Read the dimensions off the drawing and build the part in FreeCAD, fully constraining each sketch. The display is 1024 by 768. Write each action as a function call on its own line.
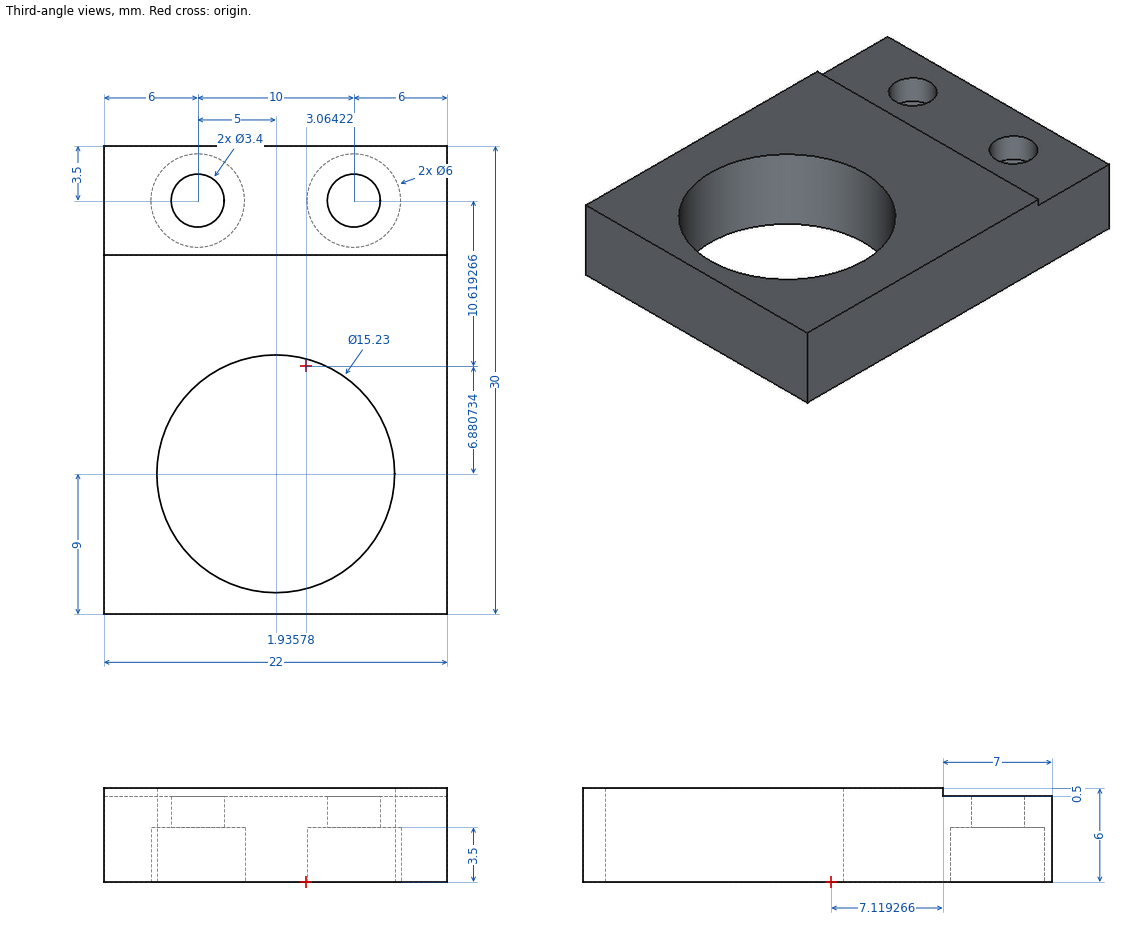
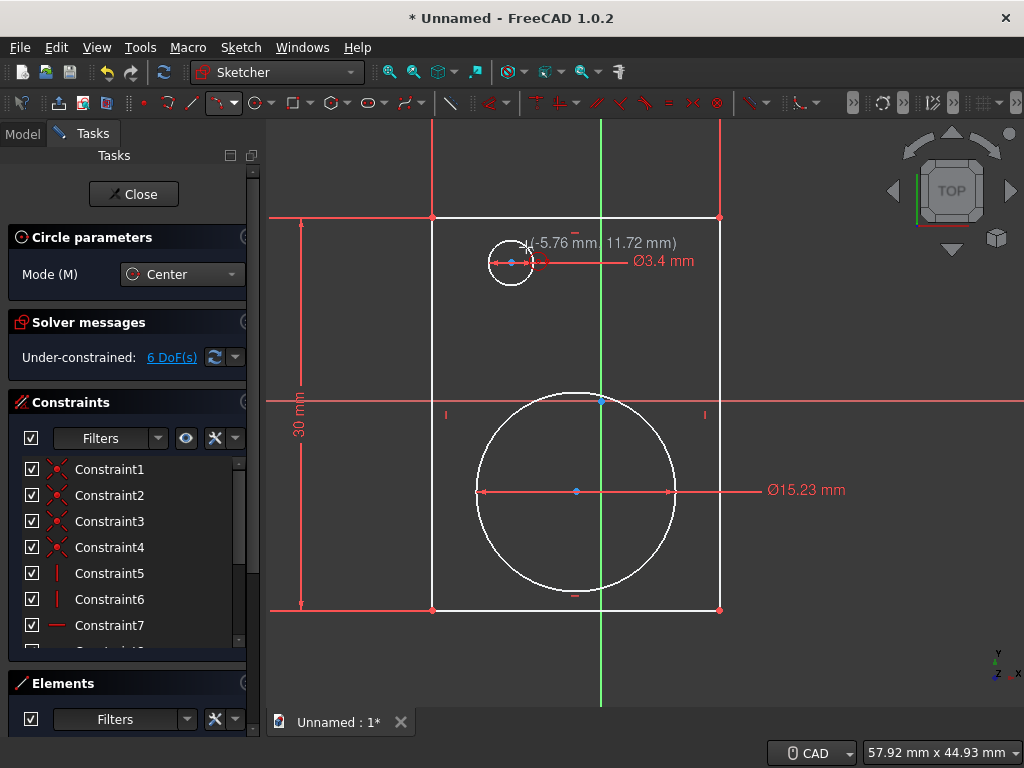
click(642, 262)
move(657, 247)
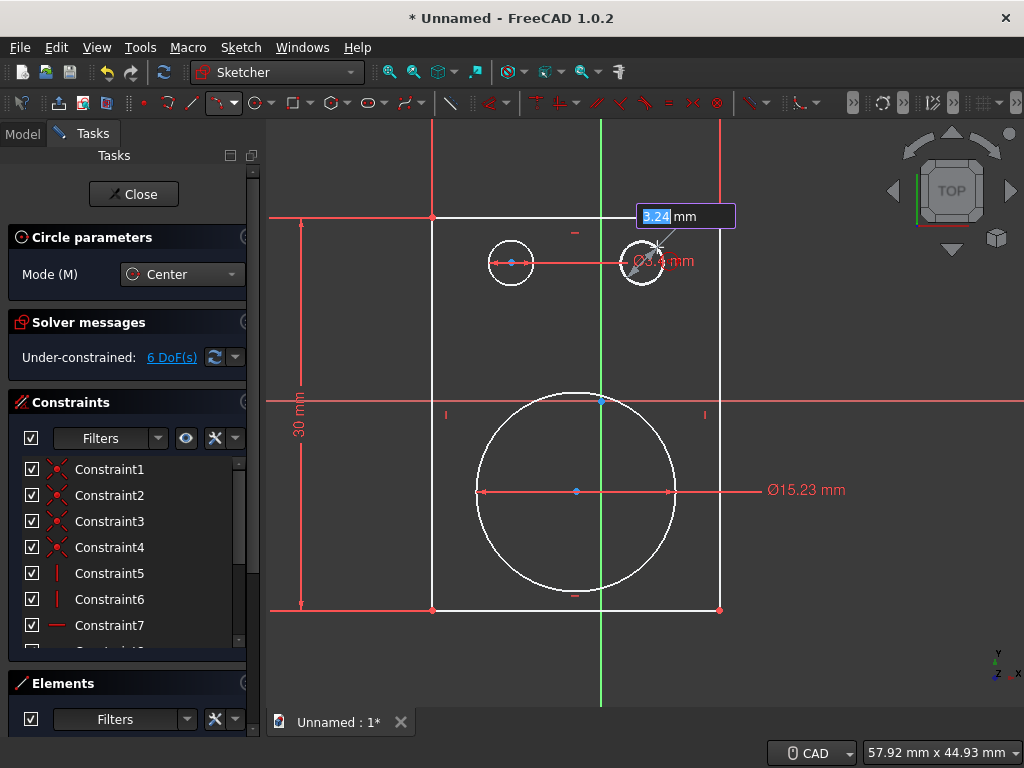
text(3.4)
key(Return)
key(Escape)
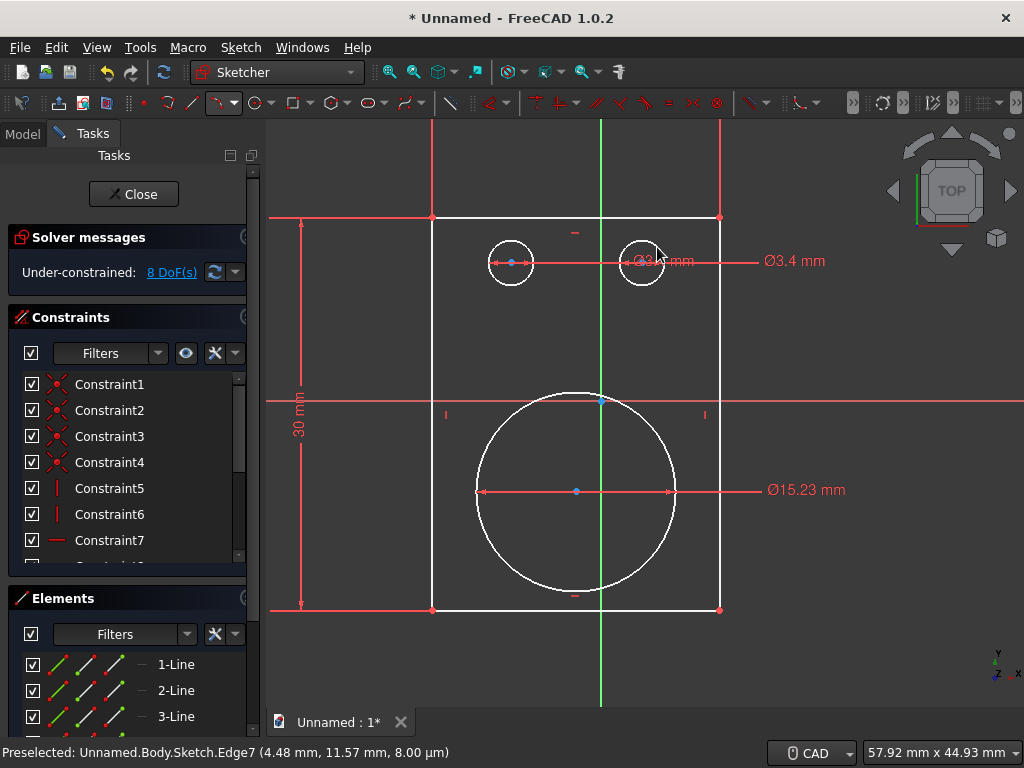
click(511, 263)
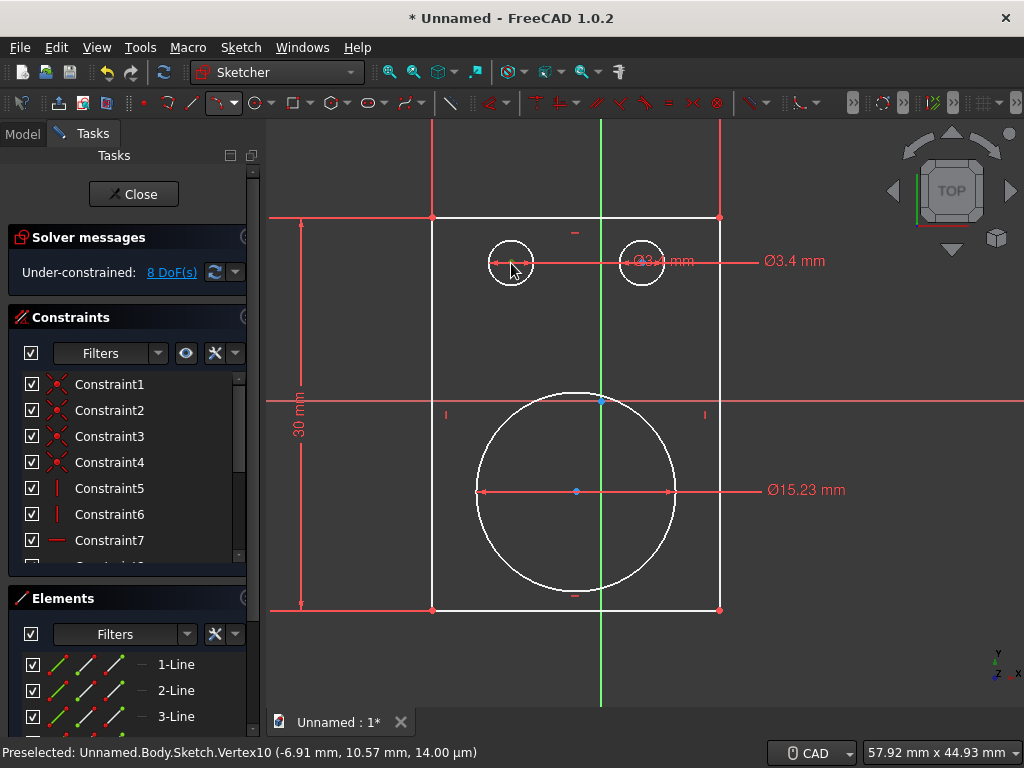
click(642, 263)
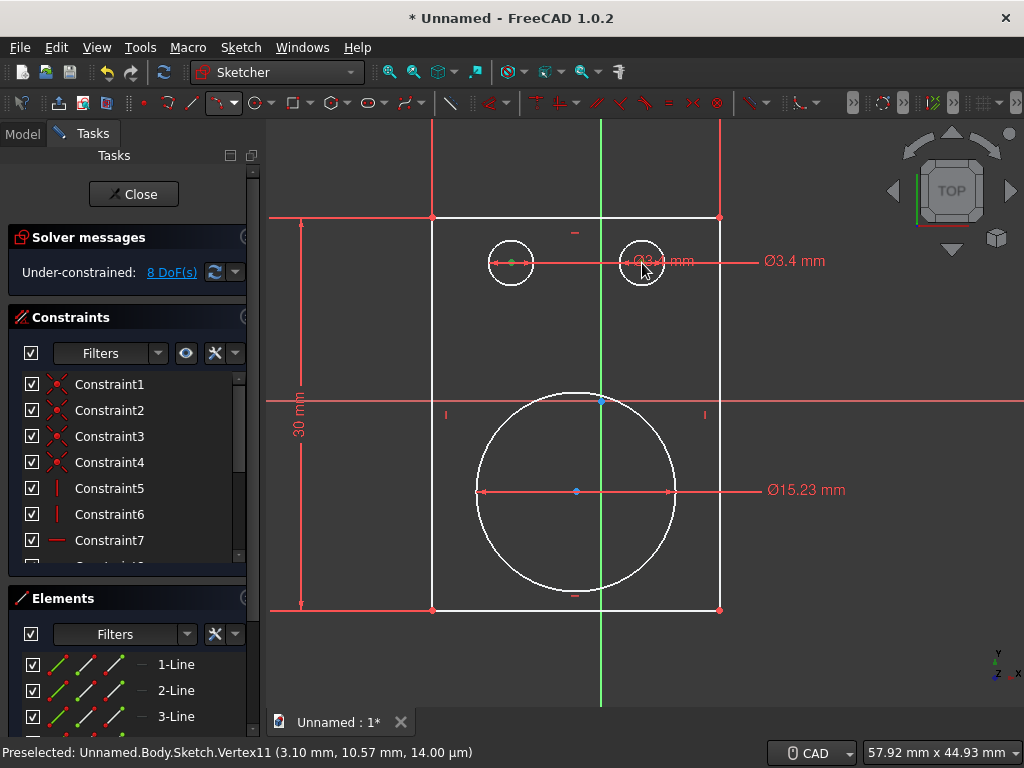
key(h)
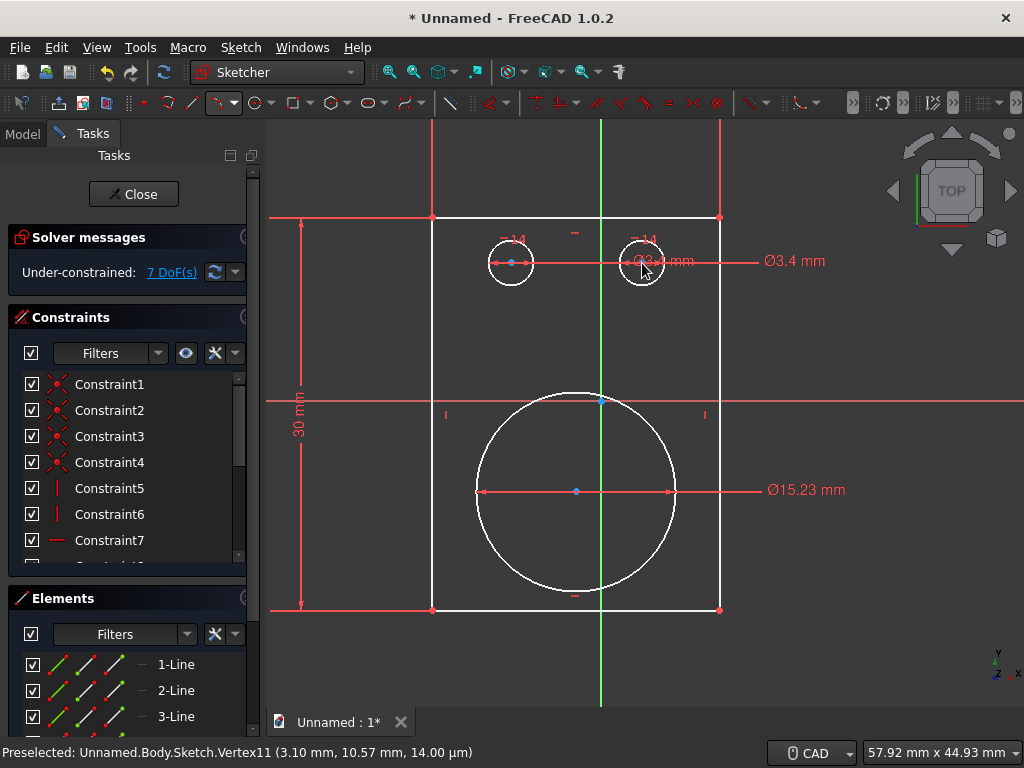
click(432, 611)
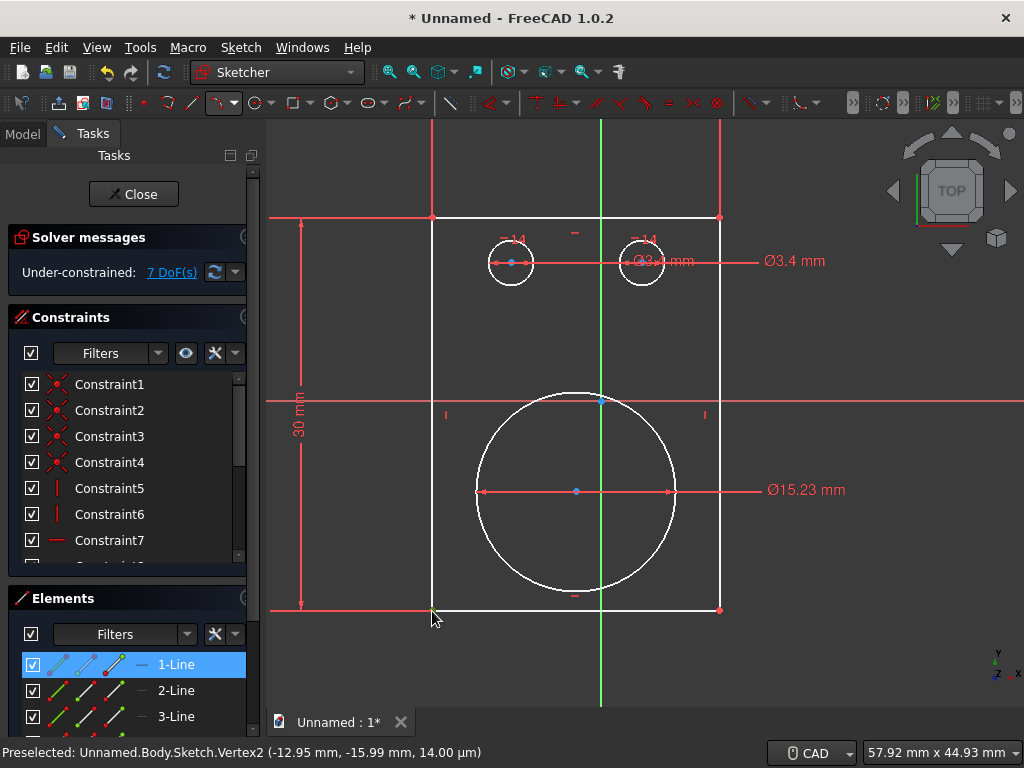
click(576, 492)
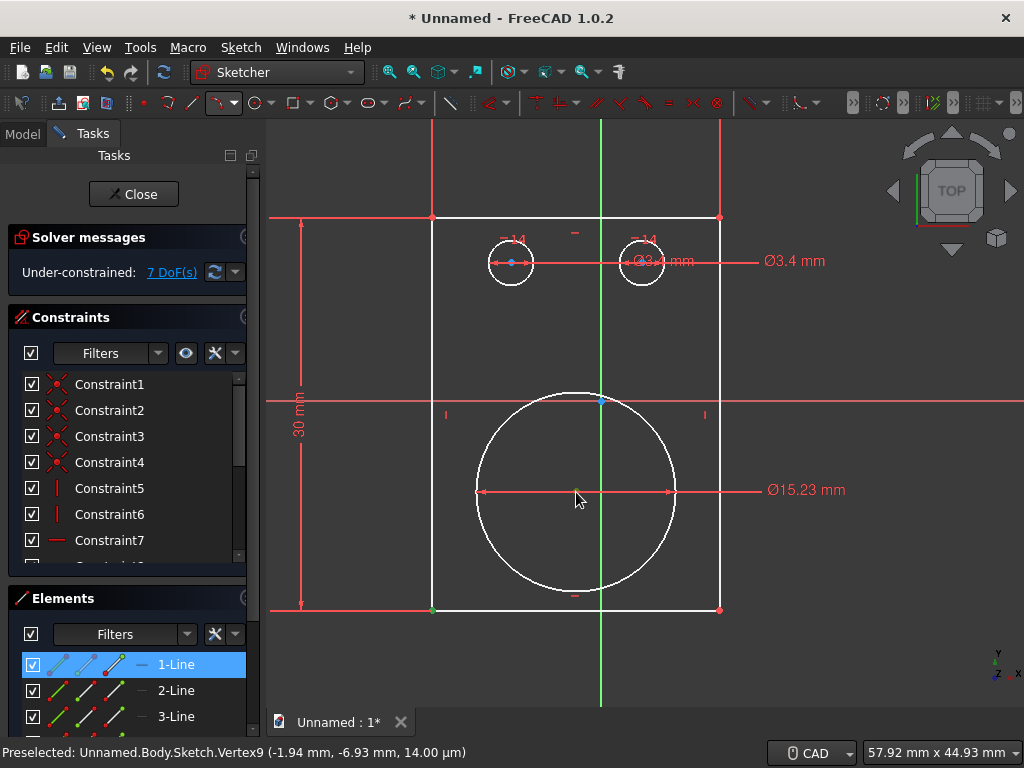
key(i)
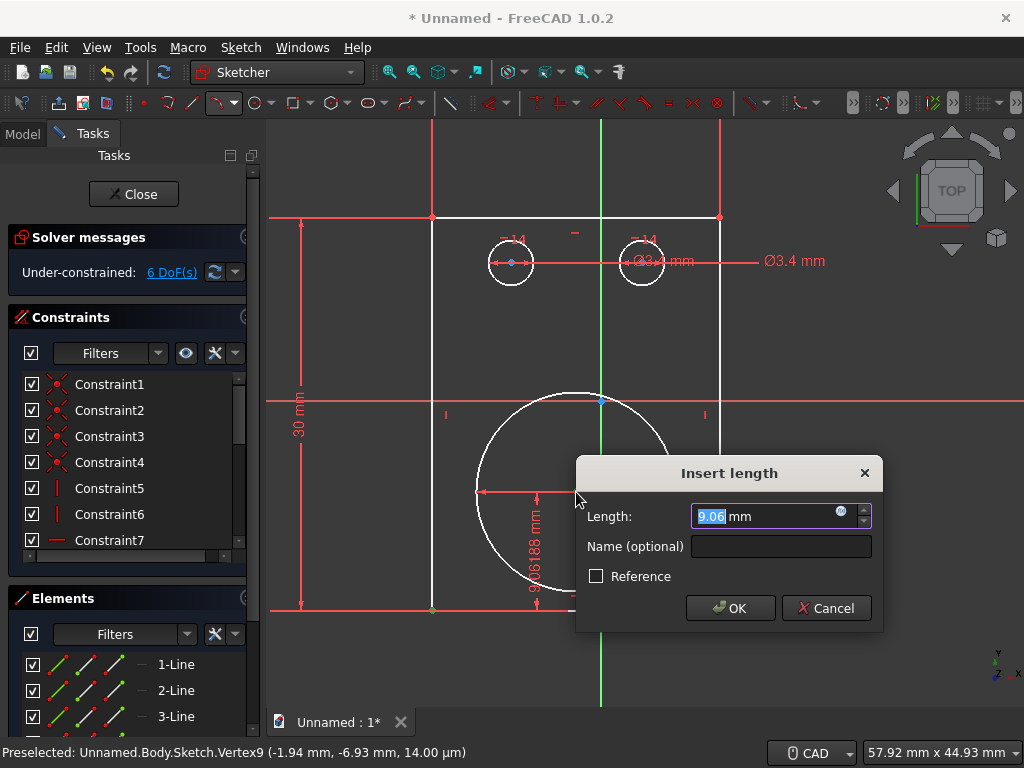
text(9)
key(Return)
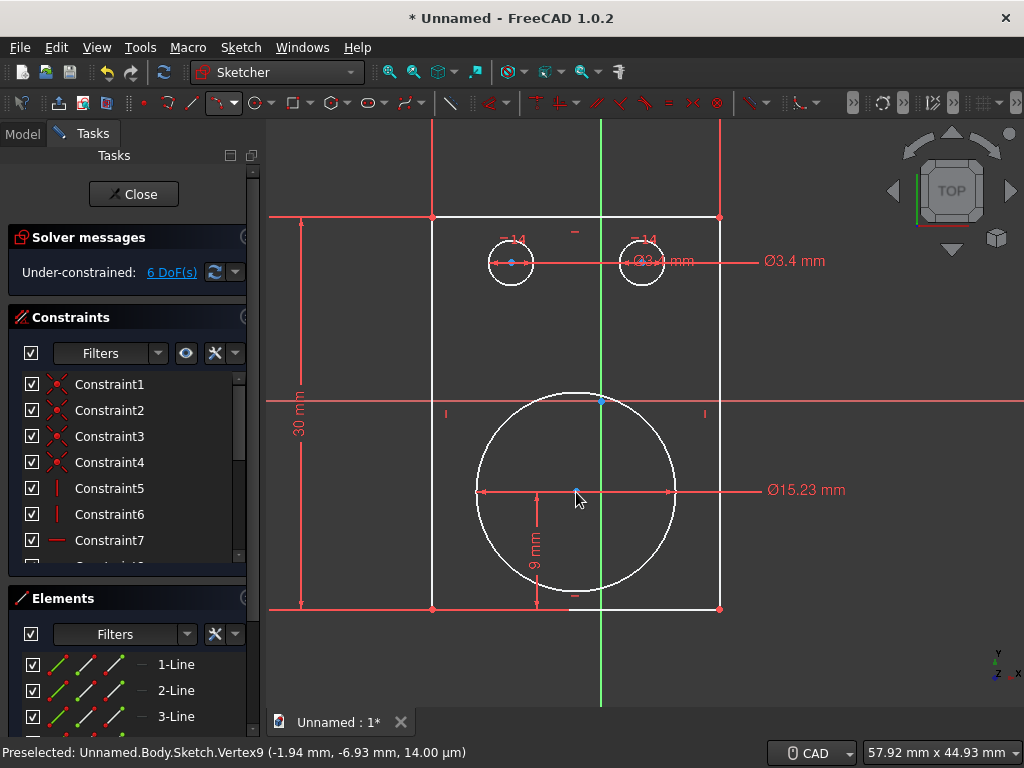
click(432, 217)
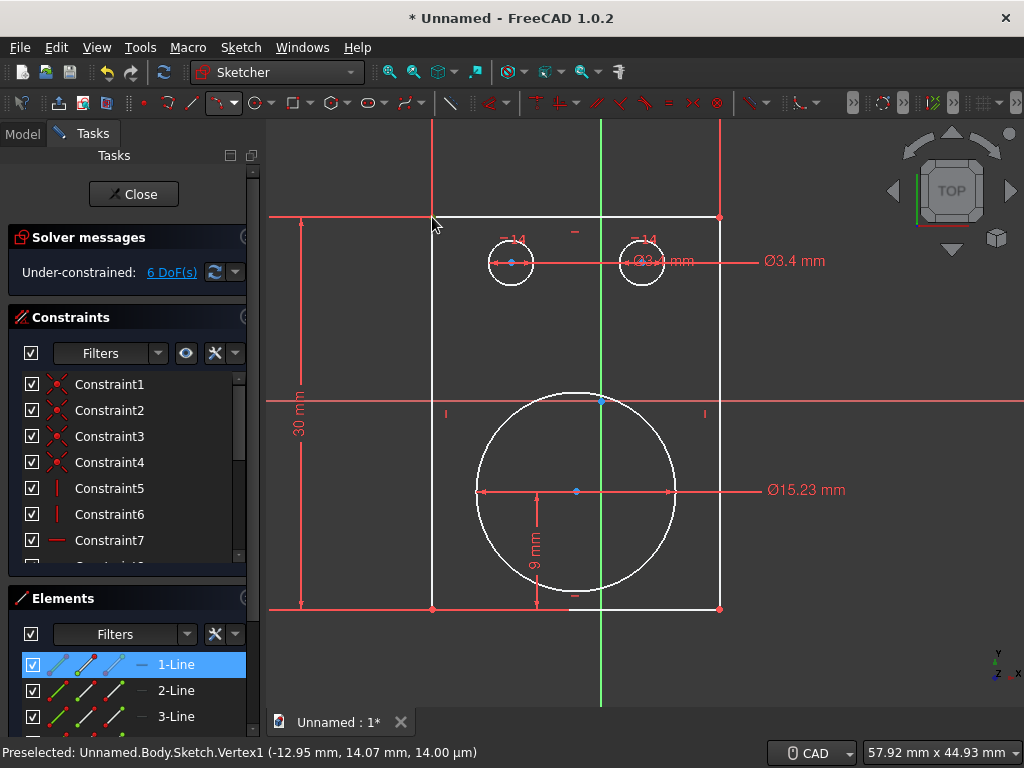
click(511, 263)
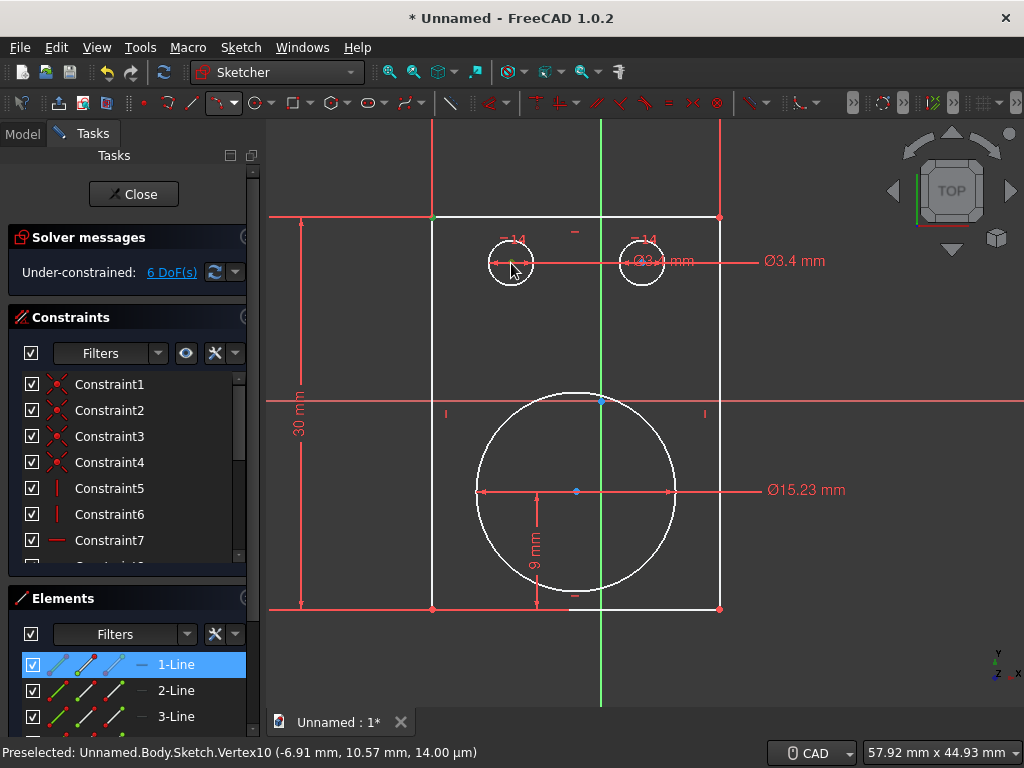
key(l)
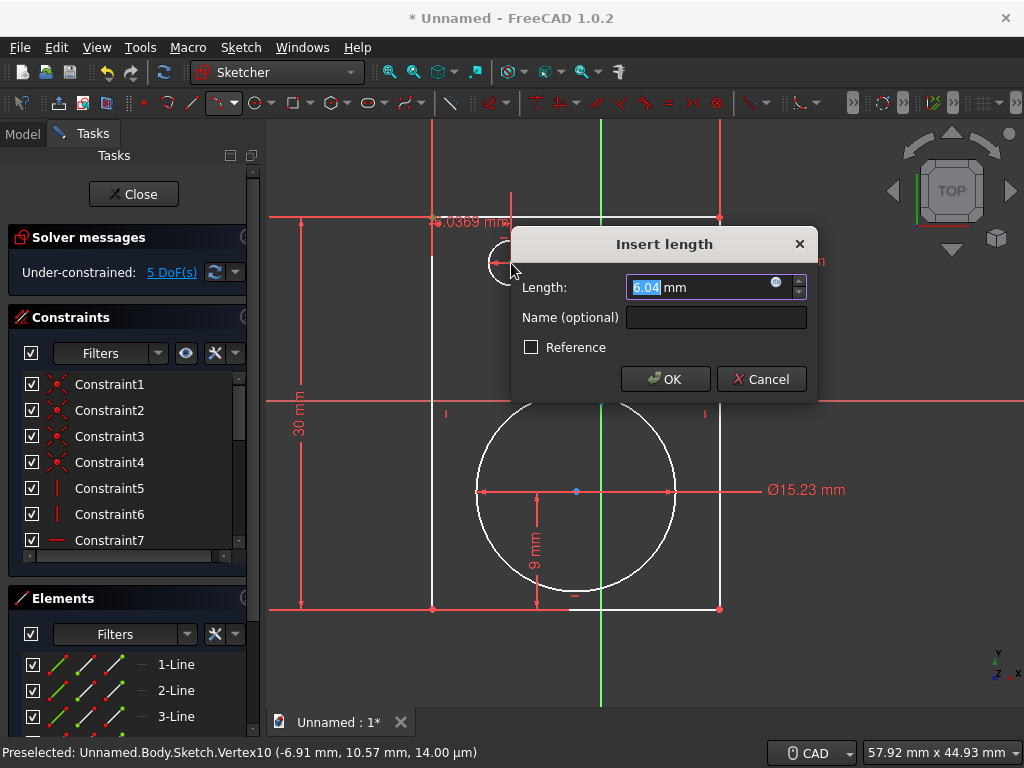
text(6)
key(Return)